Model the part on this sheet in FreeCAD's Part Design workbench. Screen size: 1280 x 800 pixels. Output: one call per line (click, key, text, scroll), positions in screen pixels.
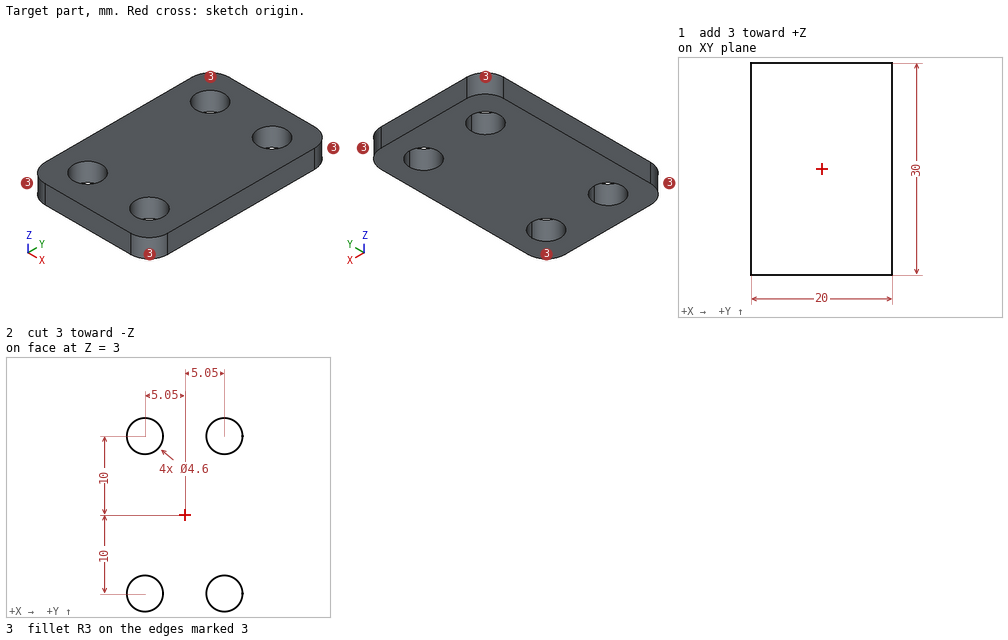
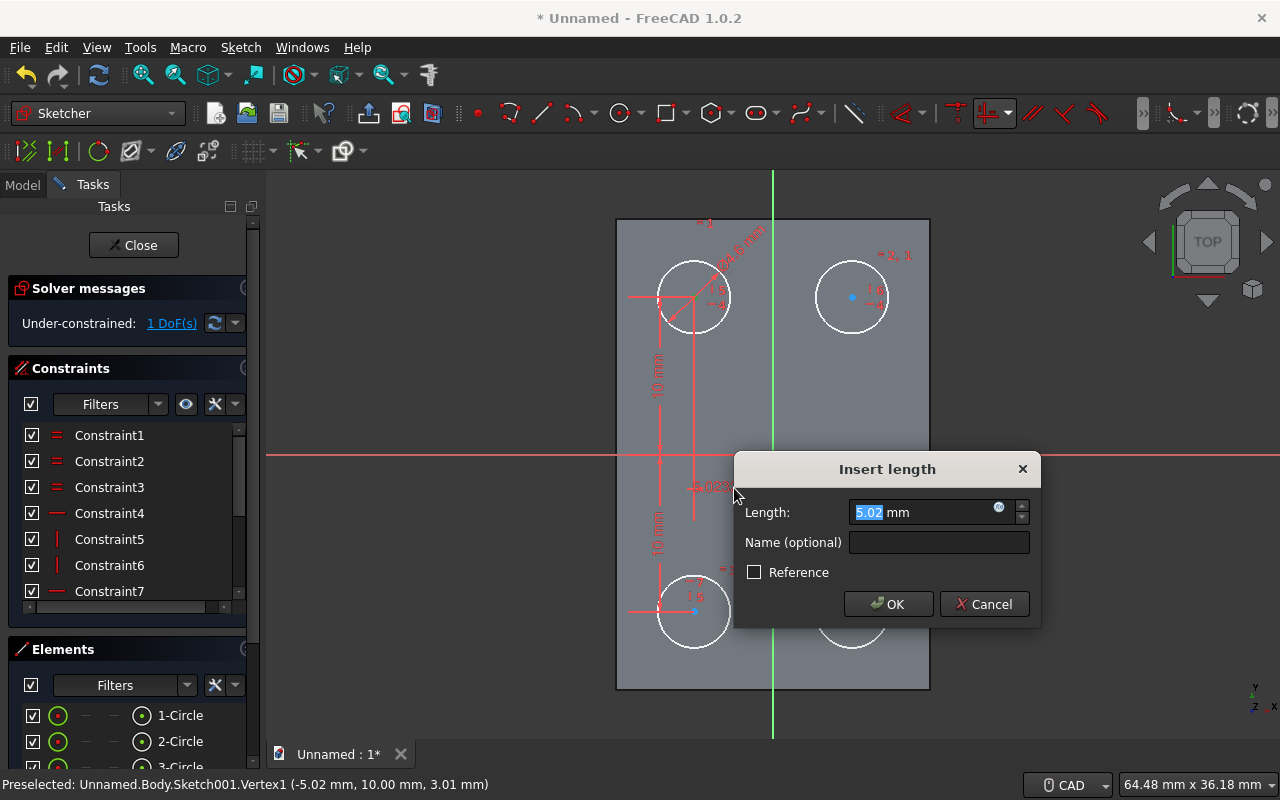
text(5.05)
key(Return)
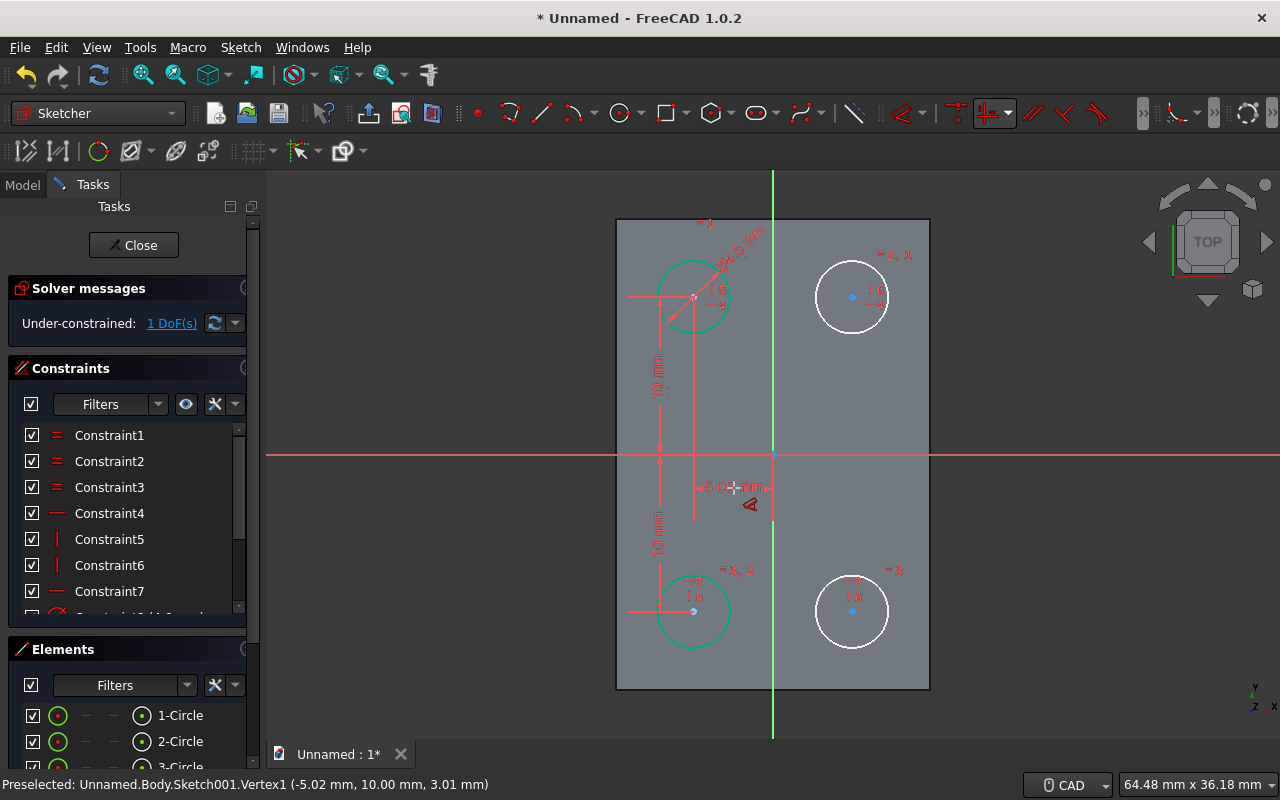
click(852, 297)
click(812, 263)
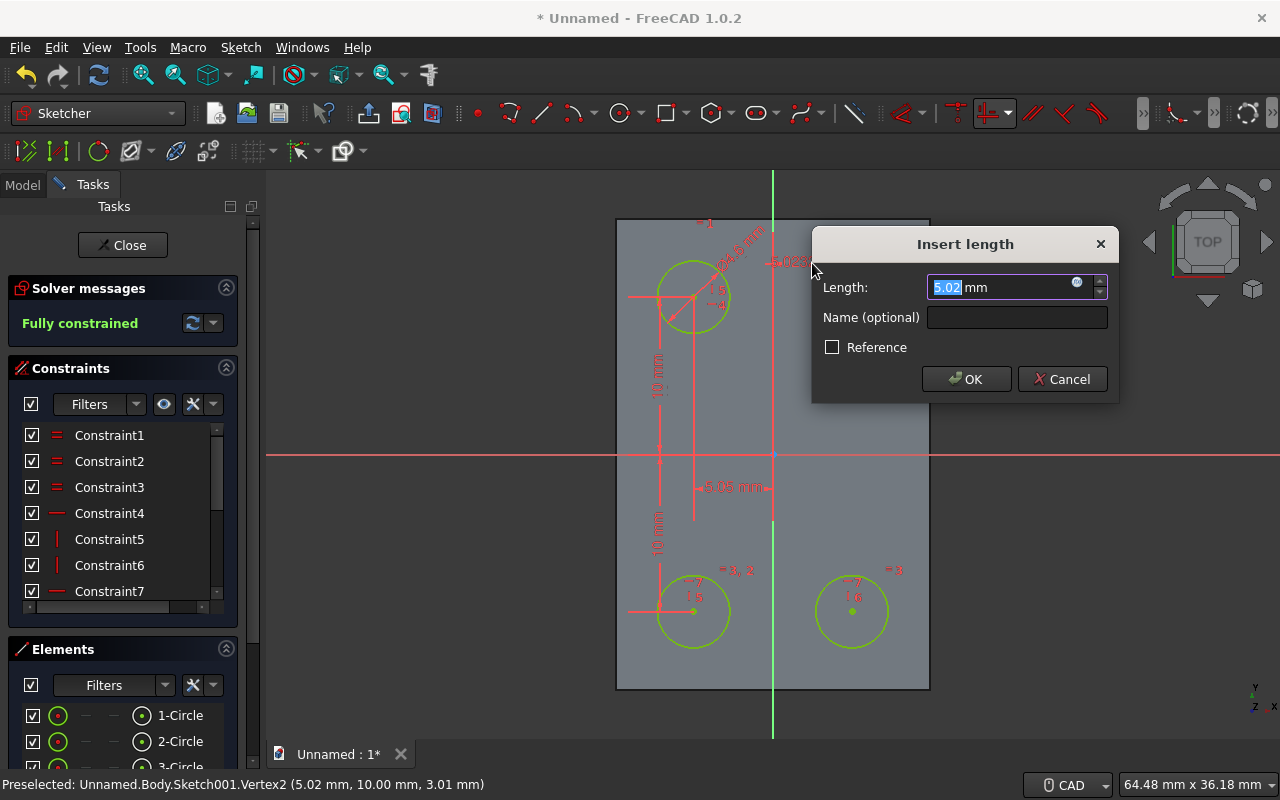
text(5.05)
key(Return)
key(Escape)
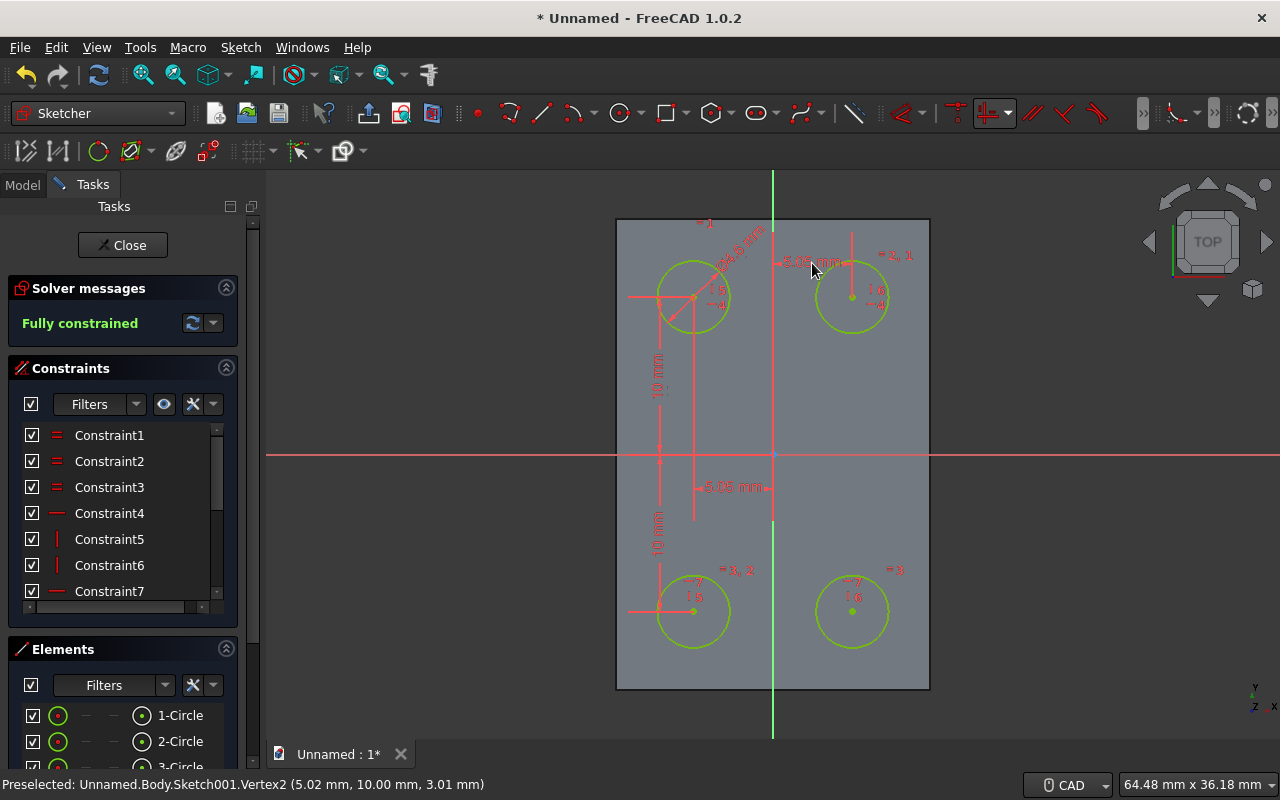
click(123, 245)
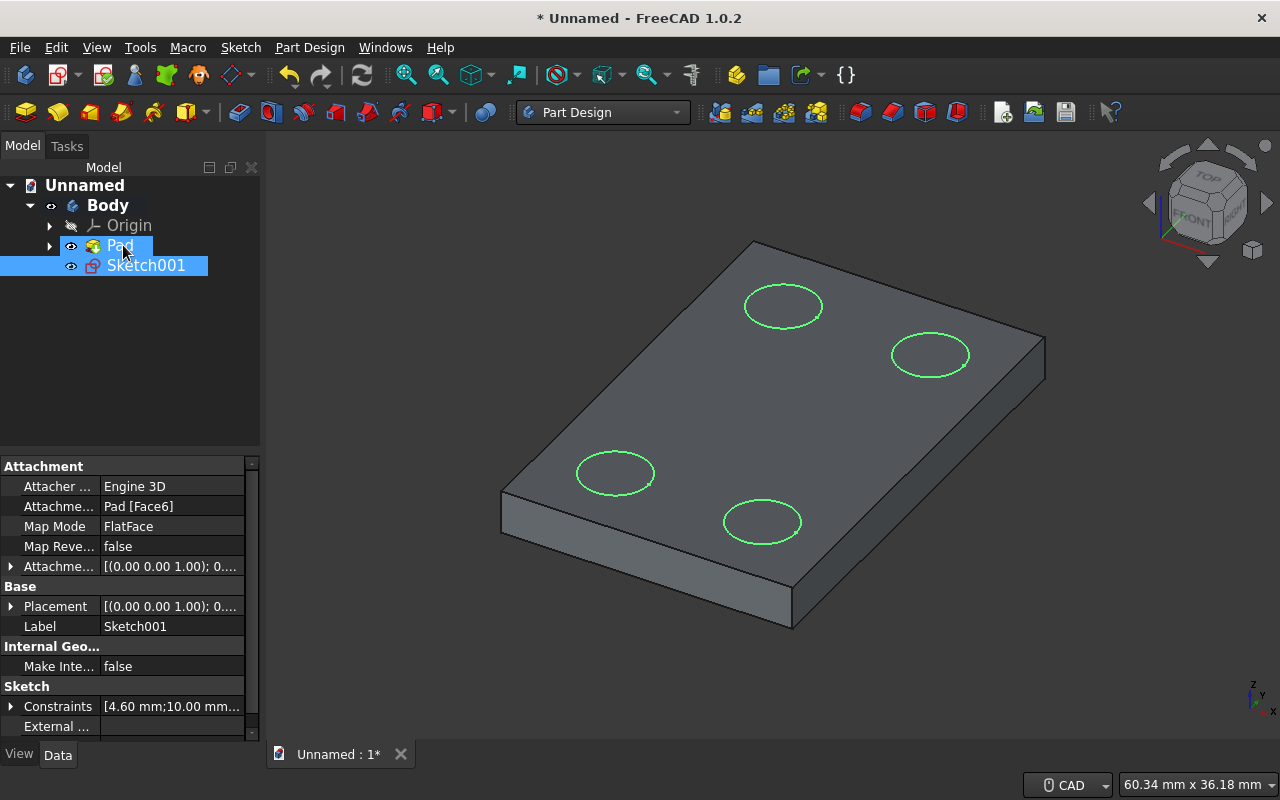
click(240, 112)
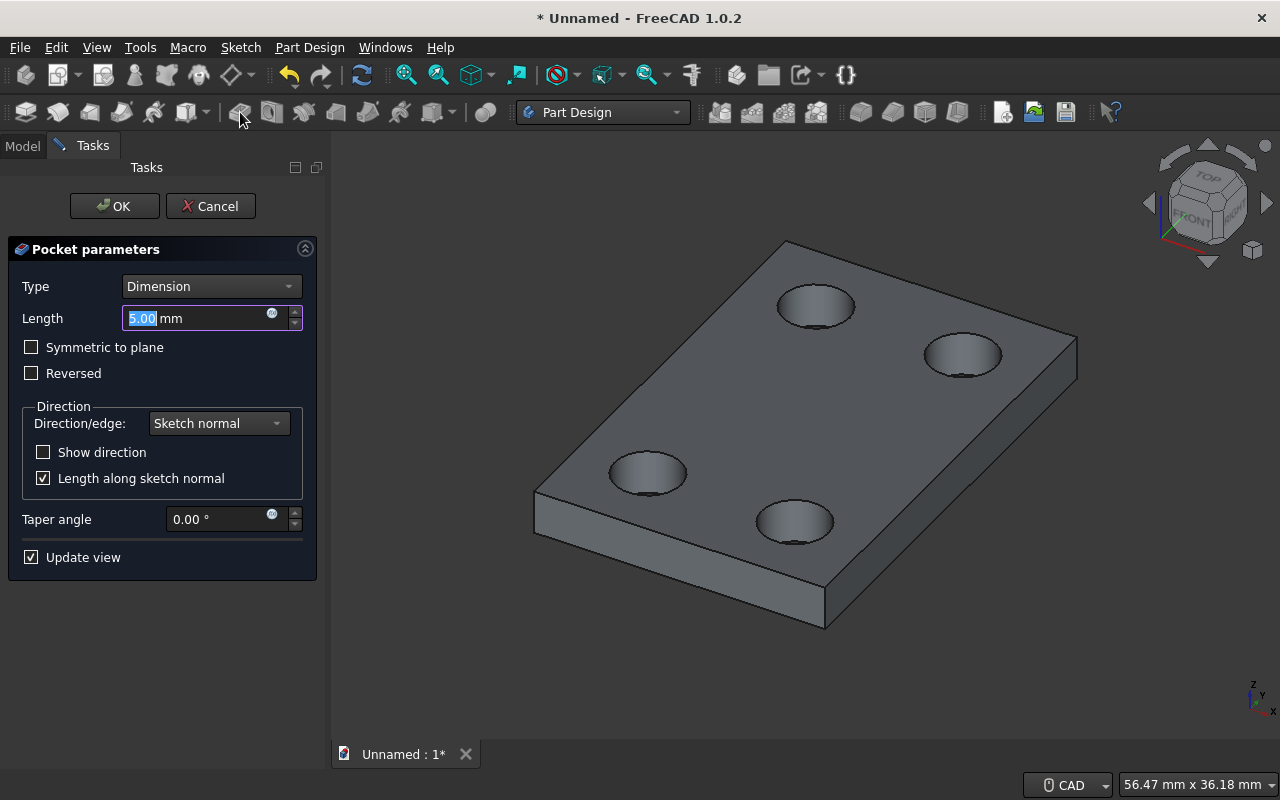
text(3)
key(Tab)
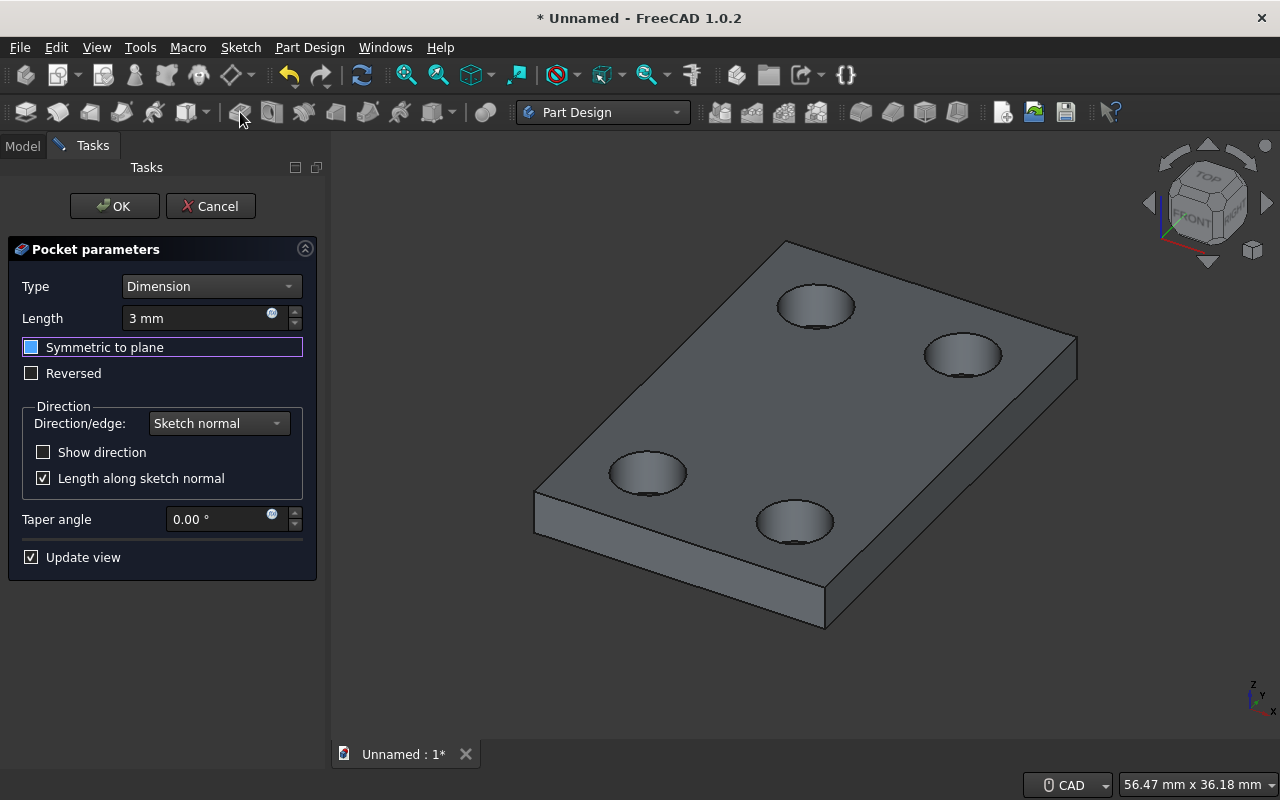
click(115, 206)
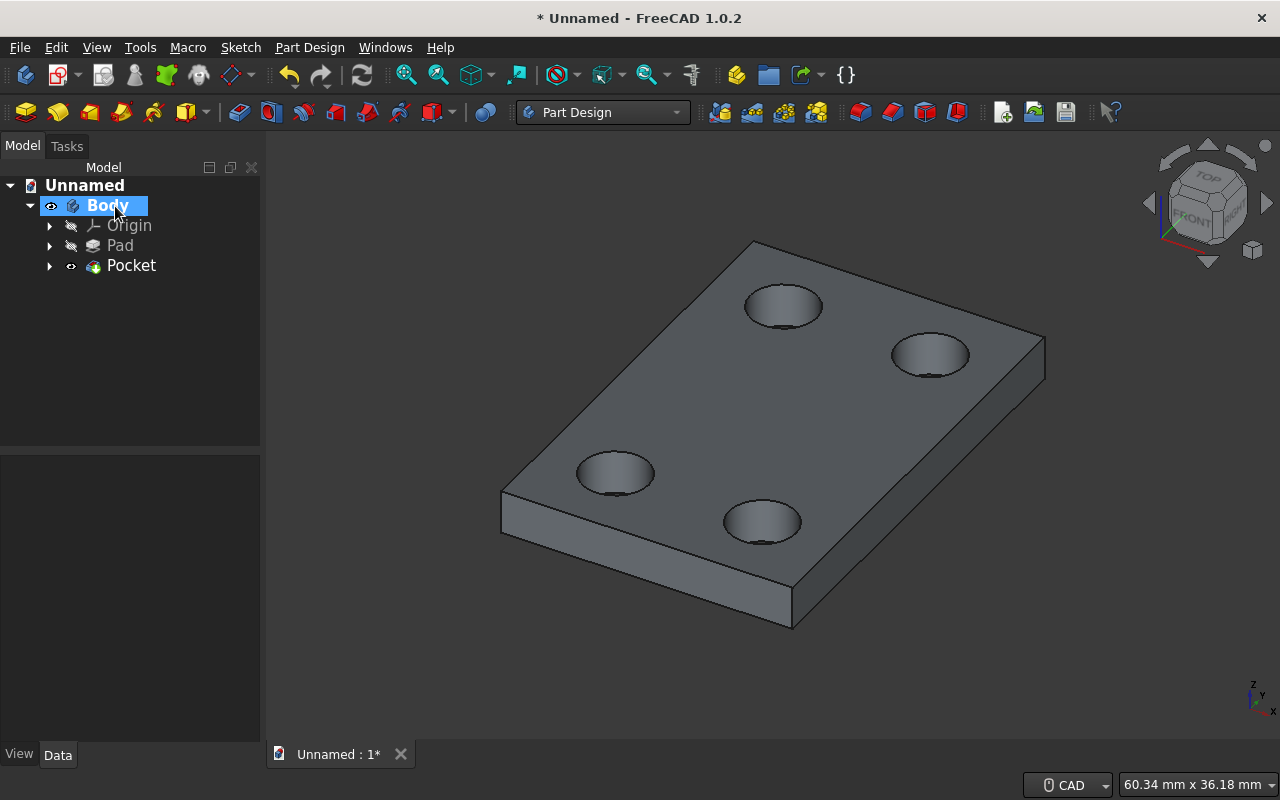
click(792, 607)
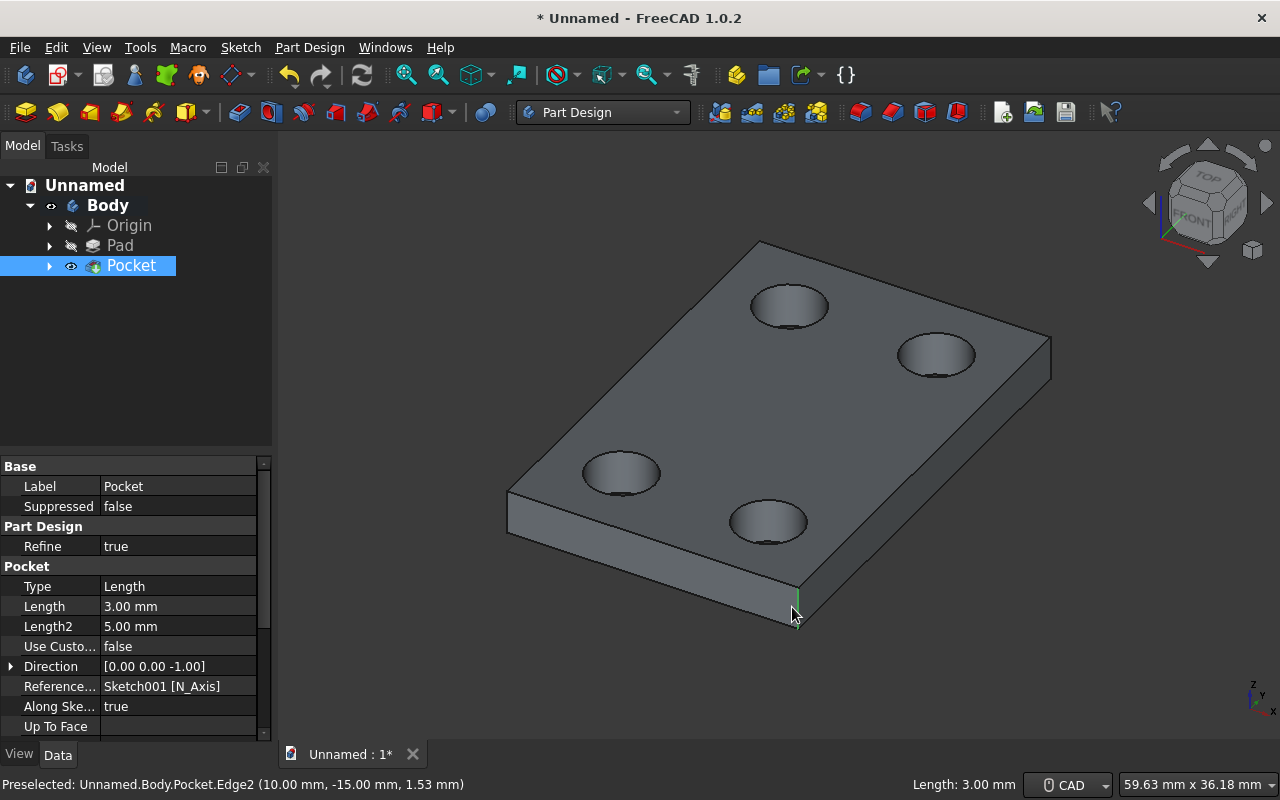
key(0)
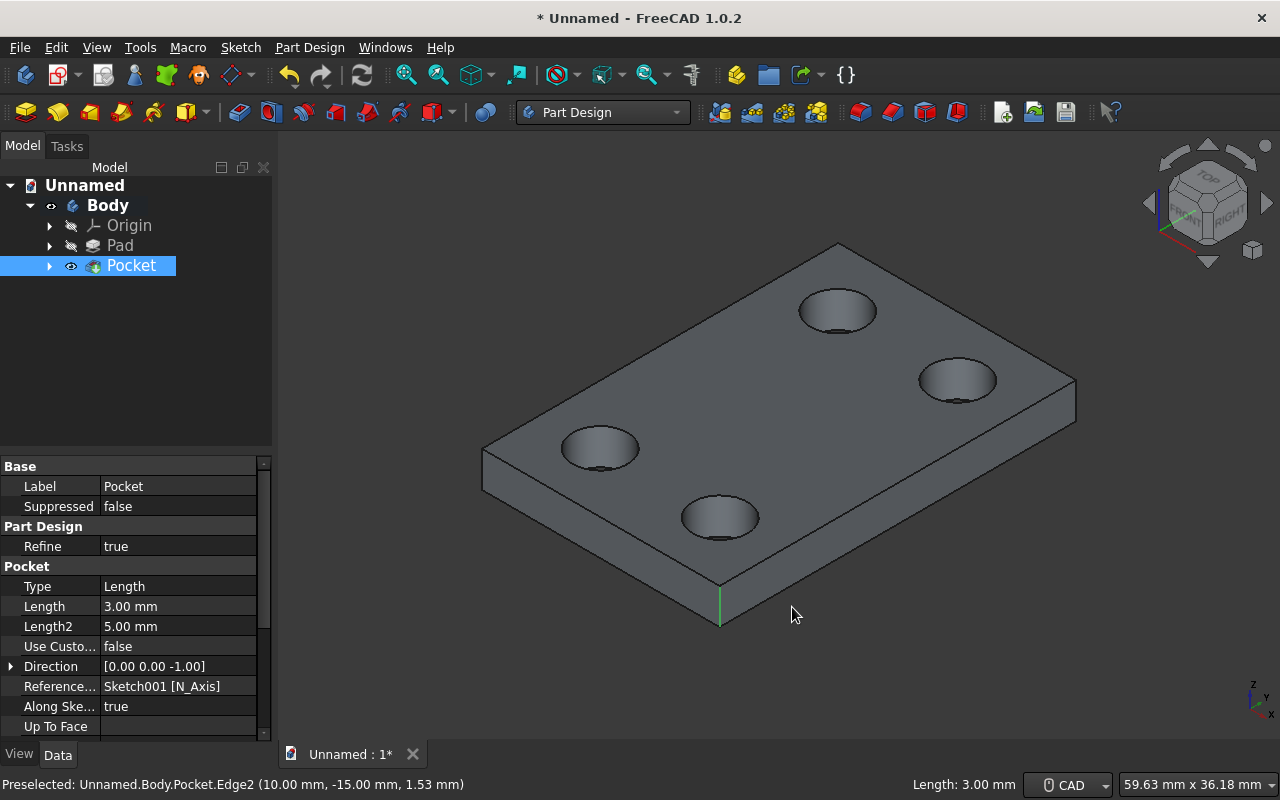
key(2)